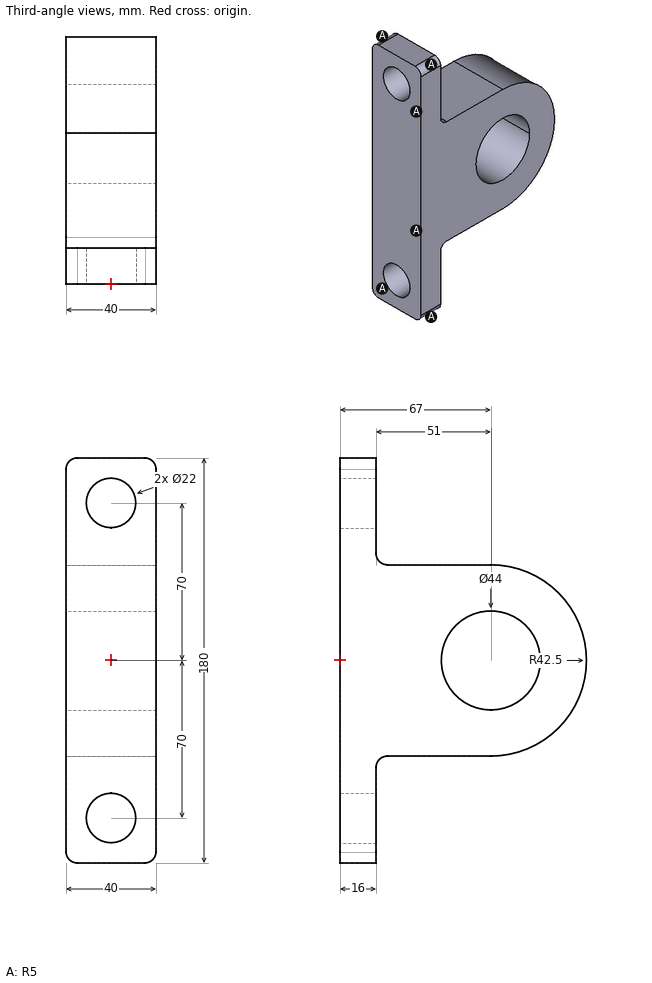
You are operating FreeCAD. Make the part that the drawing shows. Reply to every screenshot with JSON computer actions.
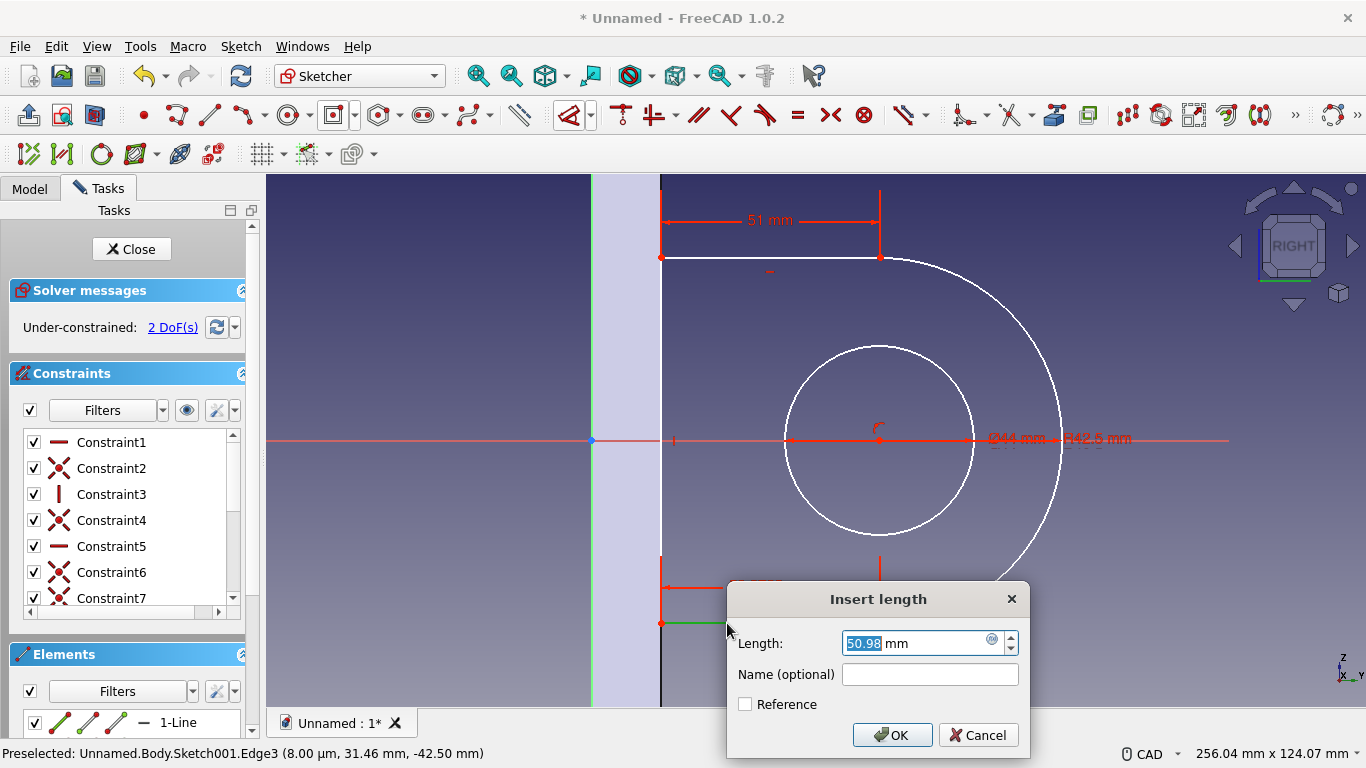
{"action": "type", "text": "51"}
{"action": "key", "text": "Return"}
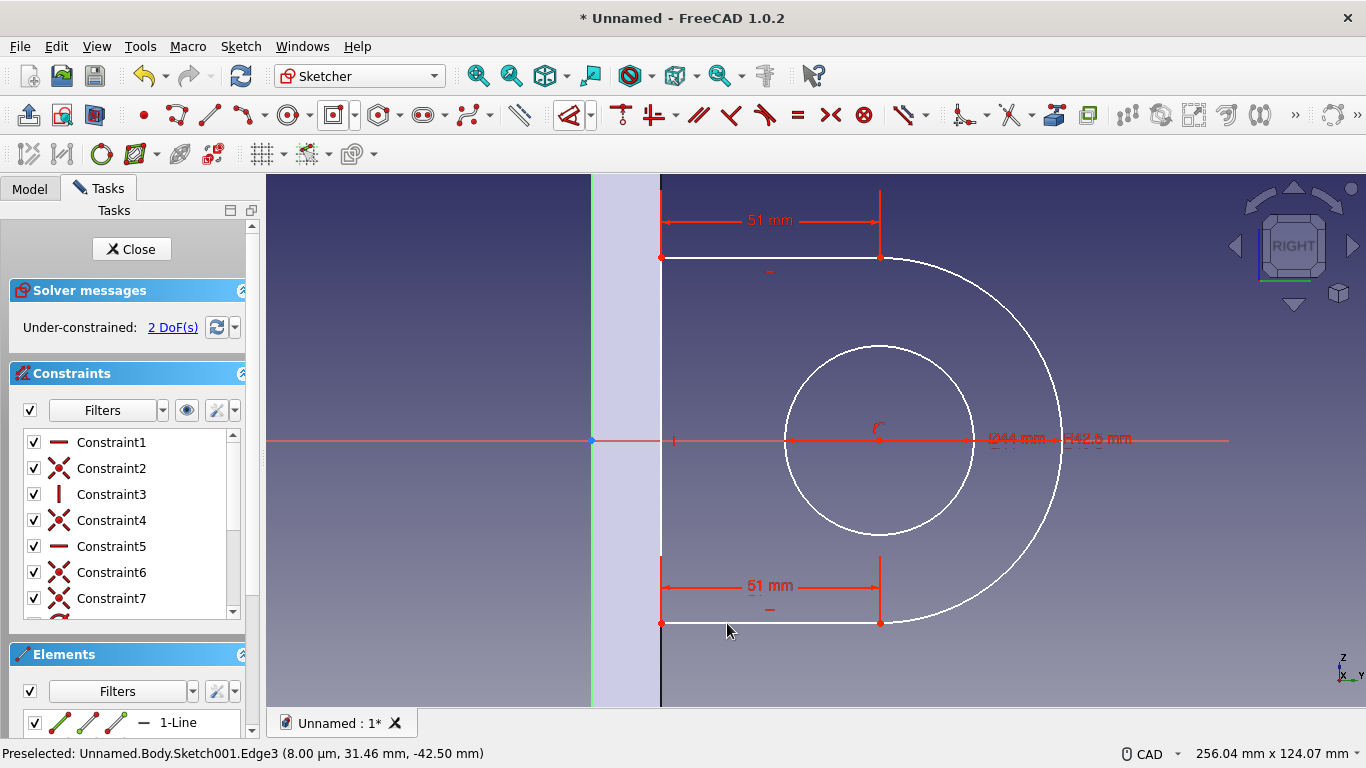
{"action": "left_click", "coordinate": [879, 440]}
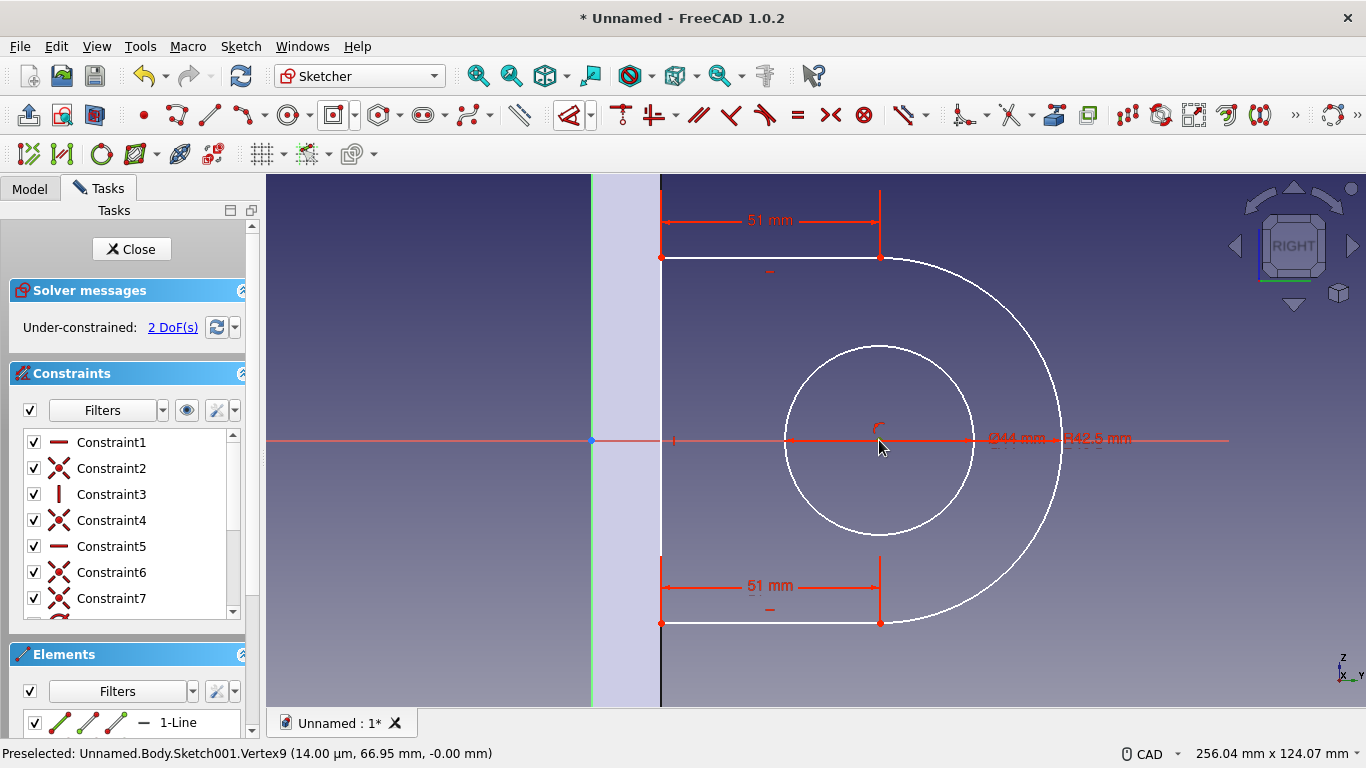
{"action": "left_click", "coordinate": [590, 116]}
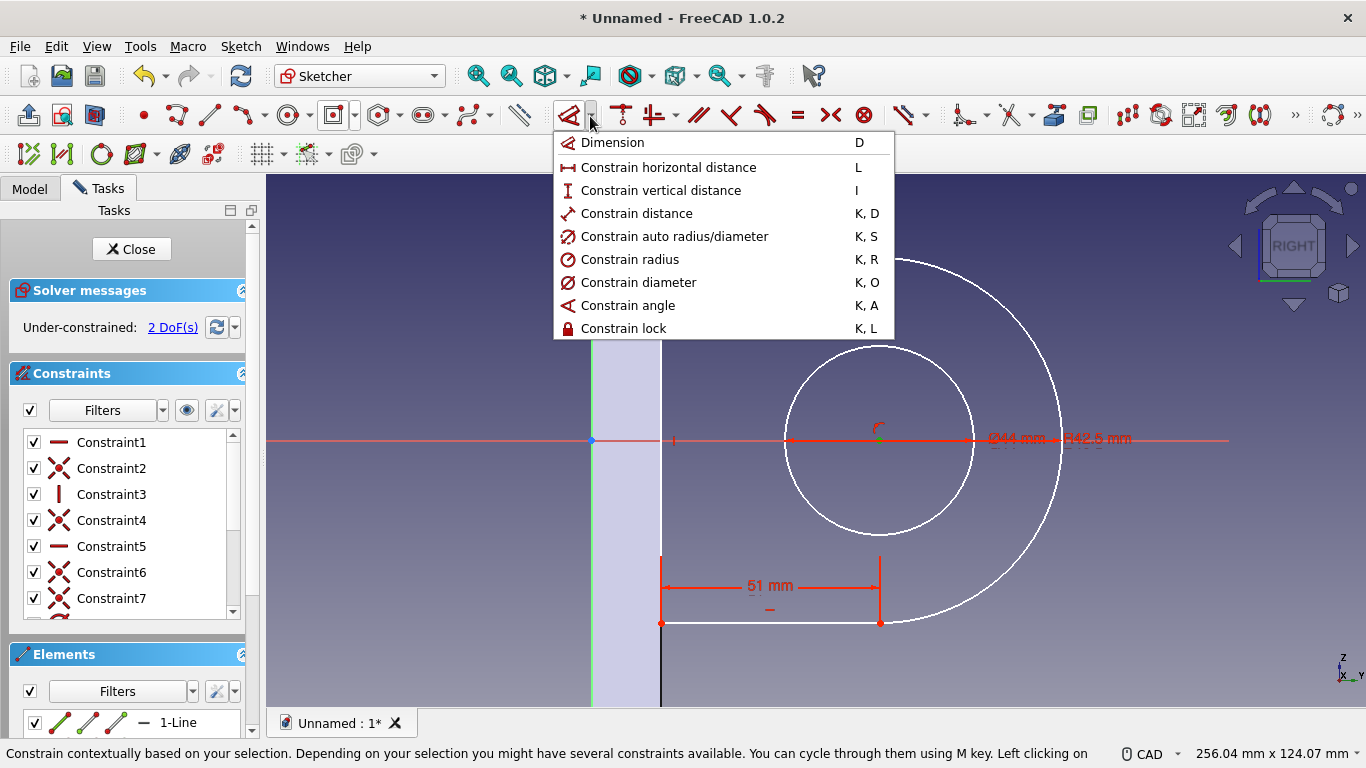
{"action": "left_click", "coordinate": [724, 168]}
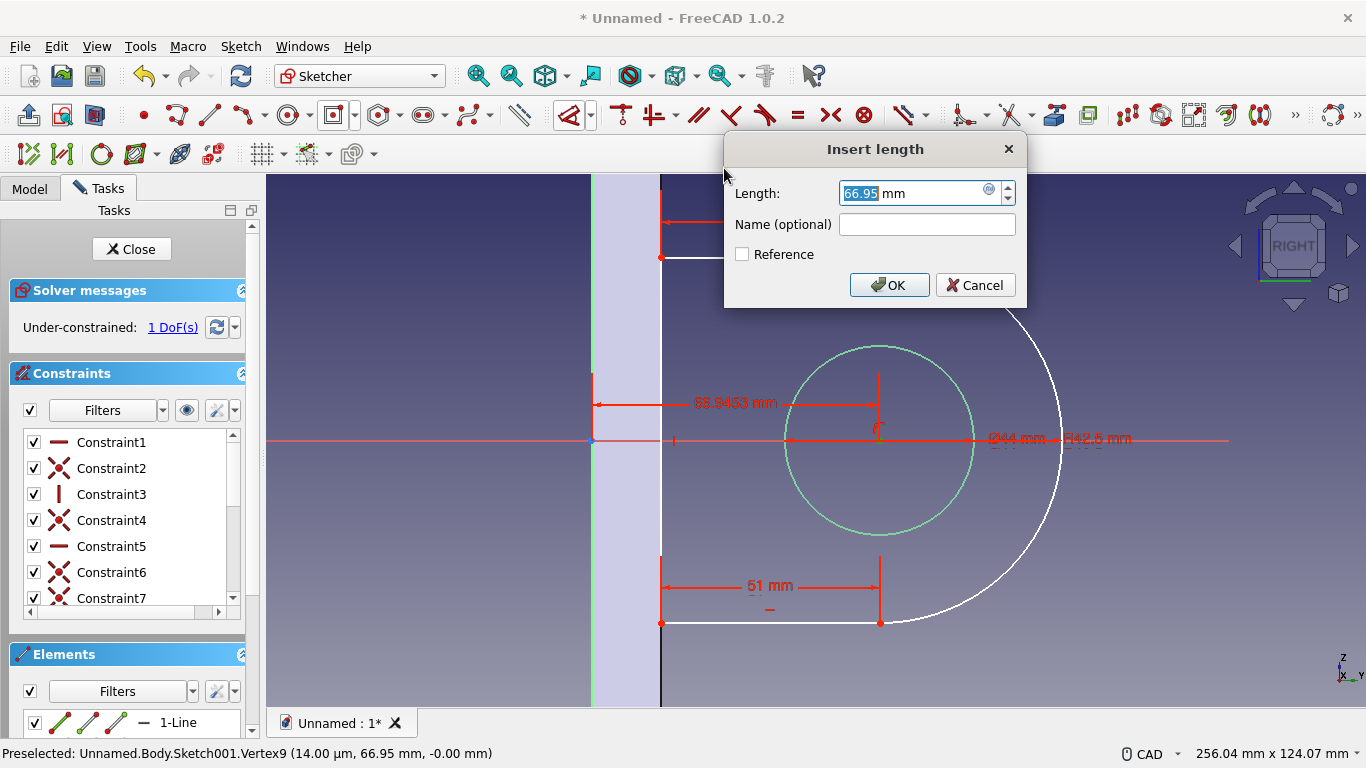
{"action": "type", "text": "67"}
{"action": "key", "text": "Return"}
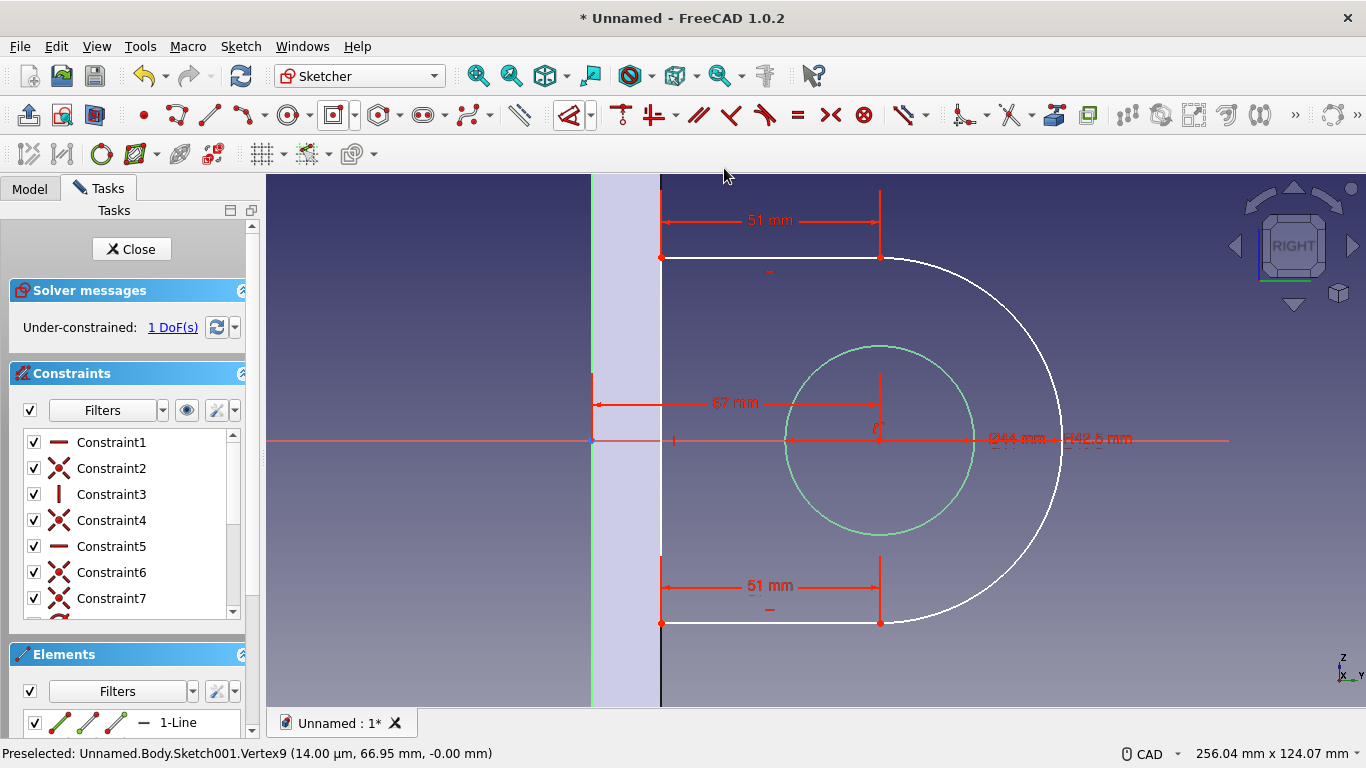
{"action": "left_click", "coordinate": [880, 258]}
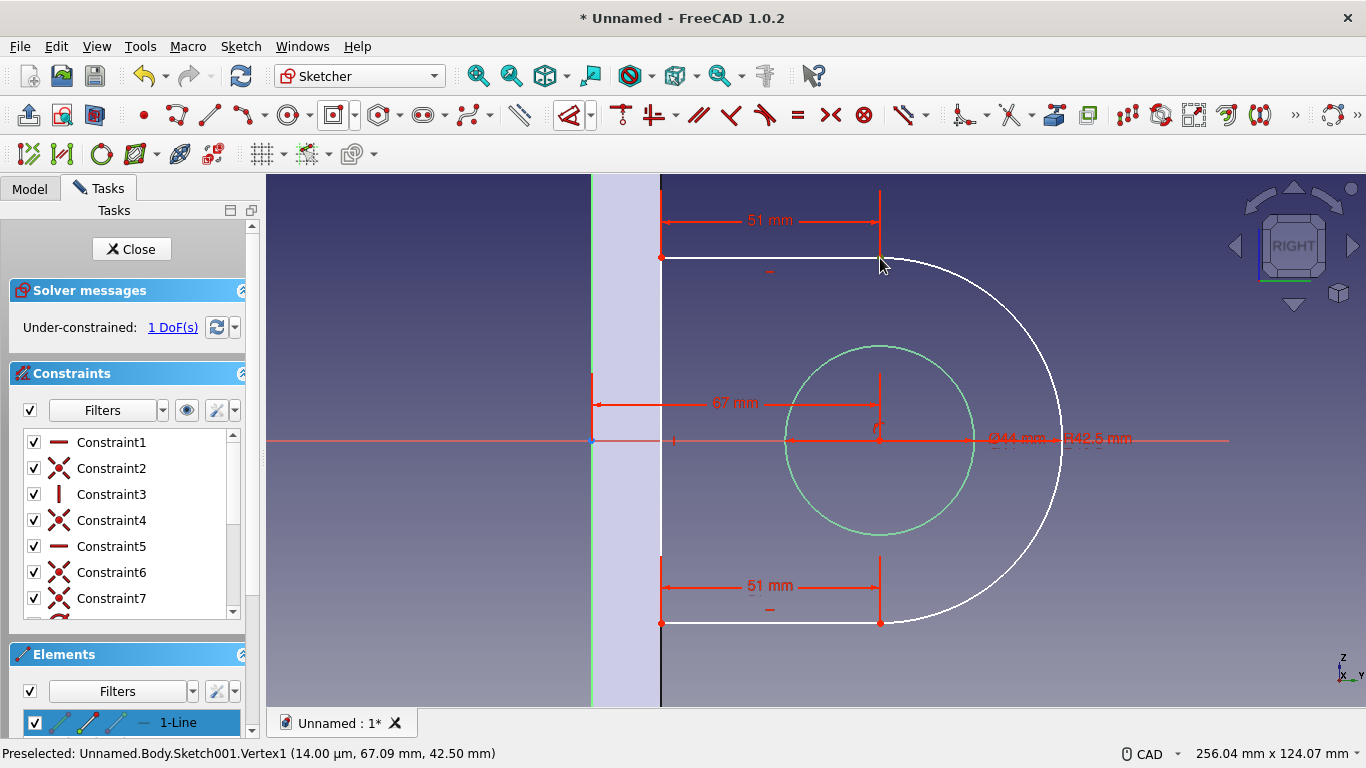
{"action": "key", "text": "l"}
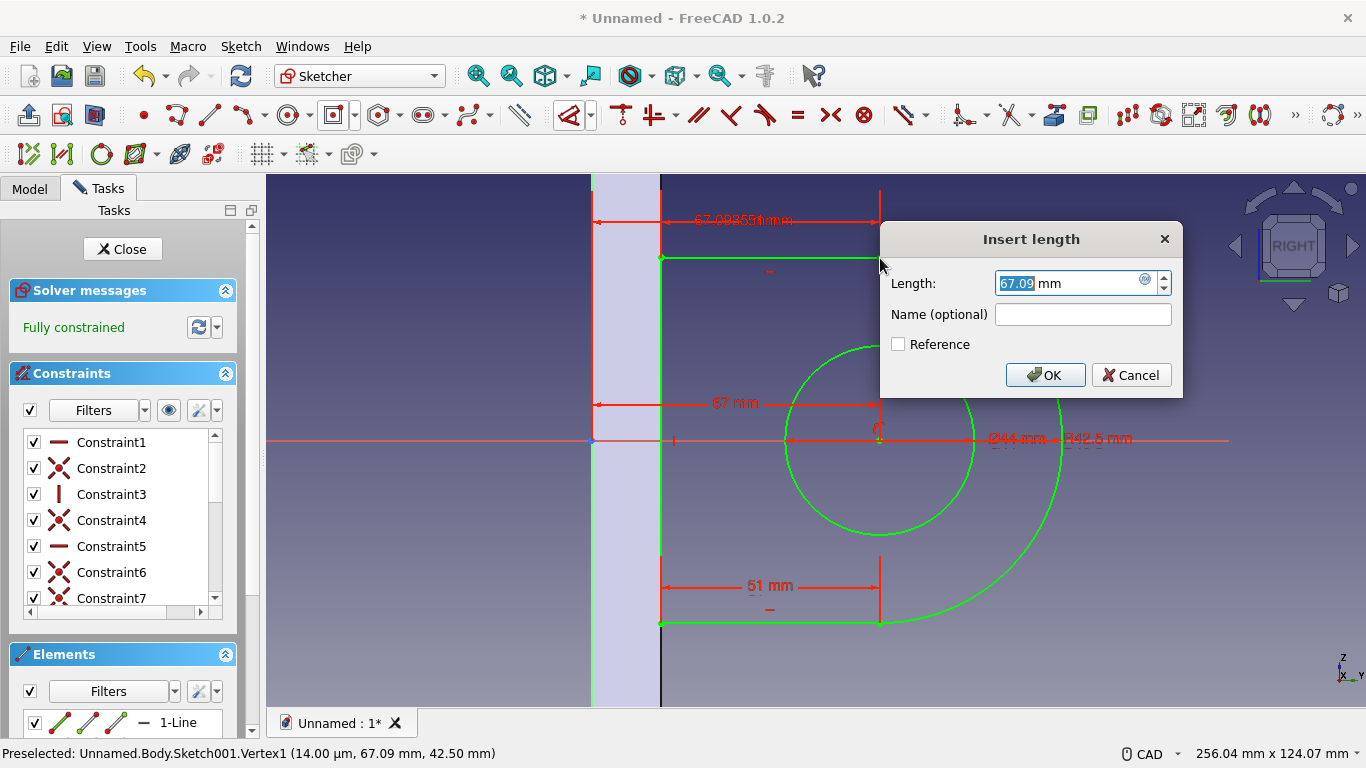
{"action": "type", "text": "67"}
{"action": "key", "text": "Return"}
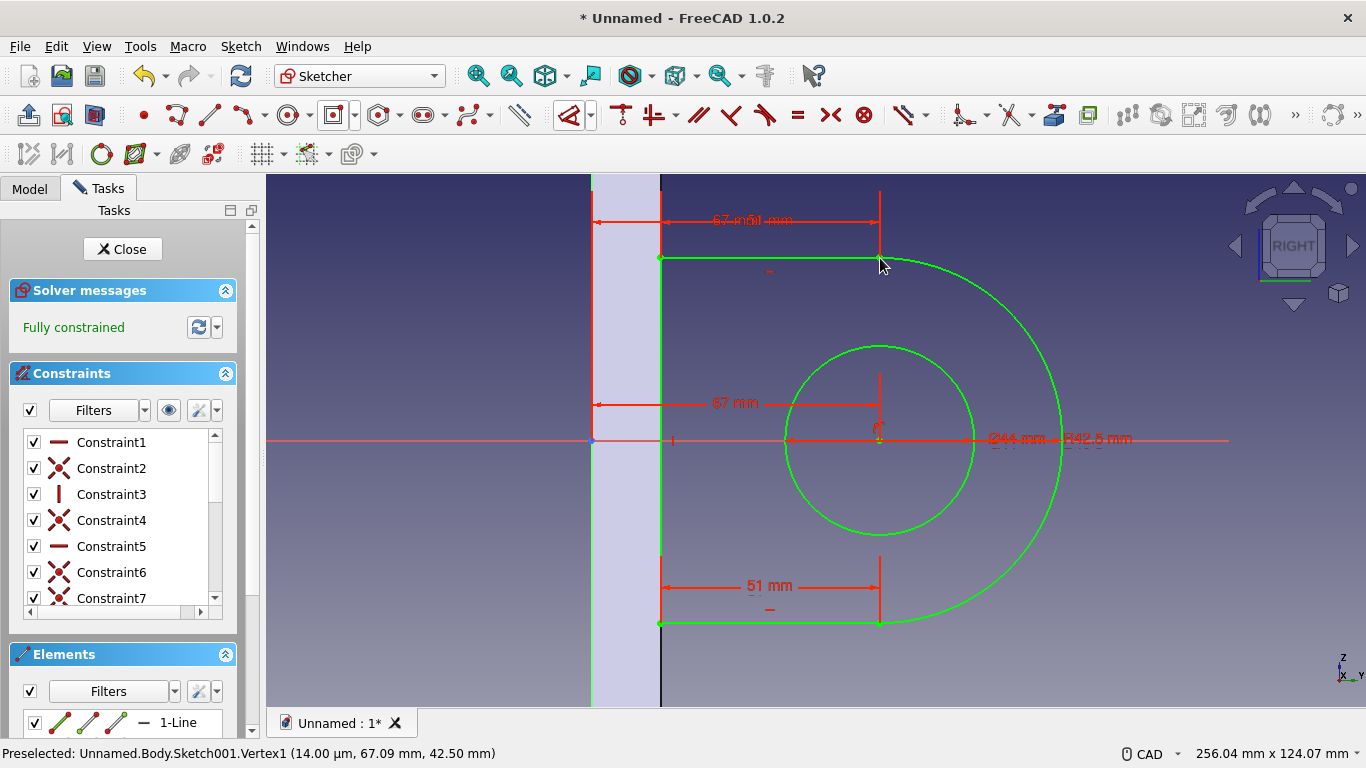
{"action": "left_click", "coordinate": [123, 249]}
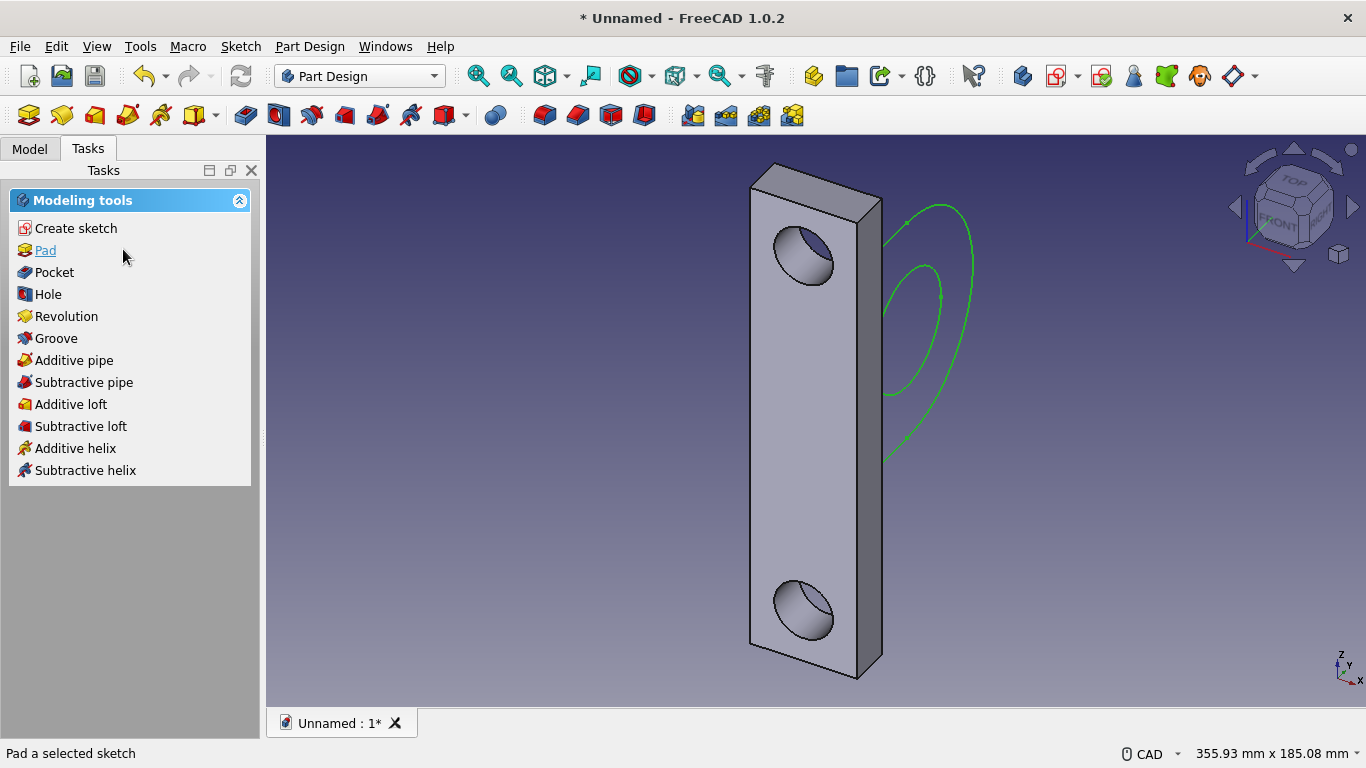
{"action": "left_click", "coordinate": [29, 116]}